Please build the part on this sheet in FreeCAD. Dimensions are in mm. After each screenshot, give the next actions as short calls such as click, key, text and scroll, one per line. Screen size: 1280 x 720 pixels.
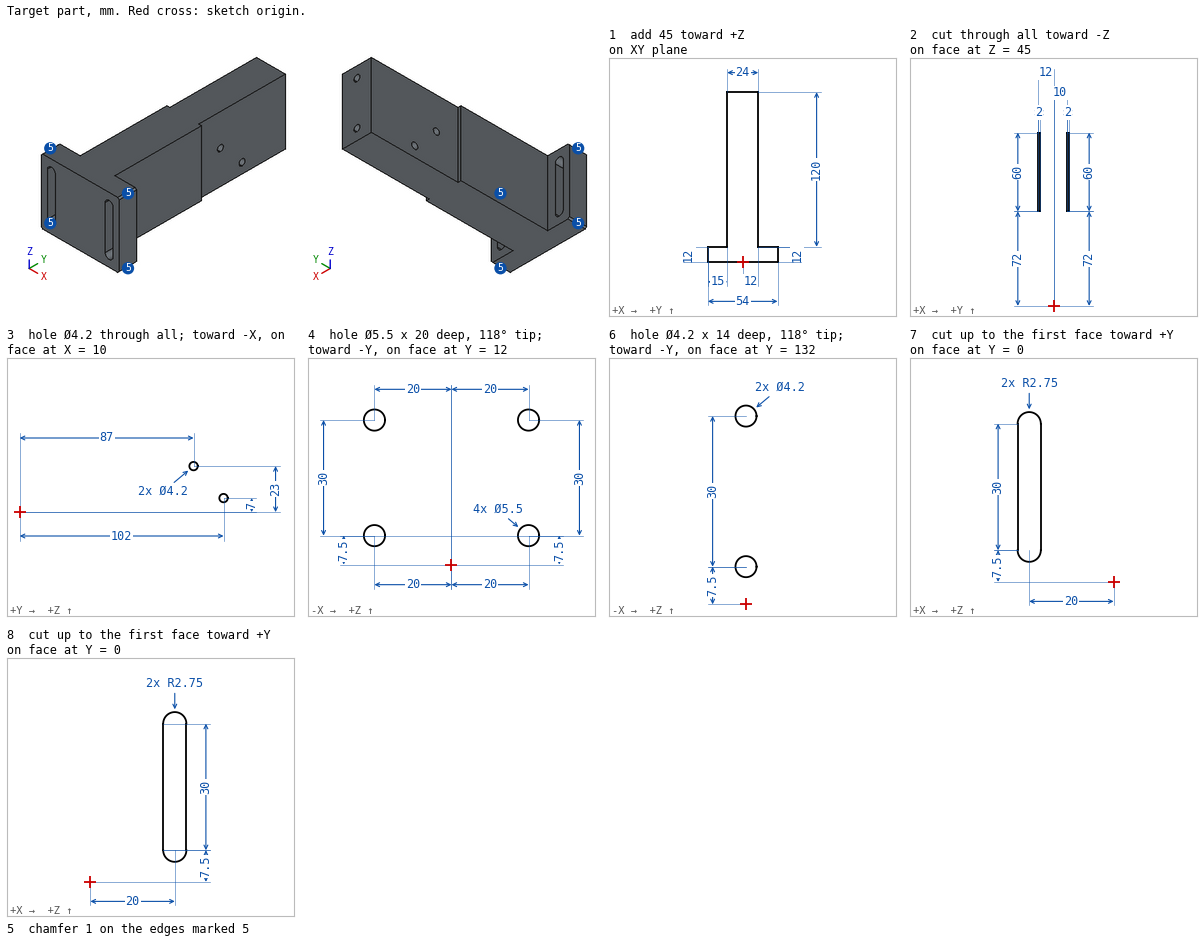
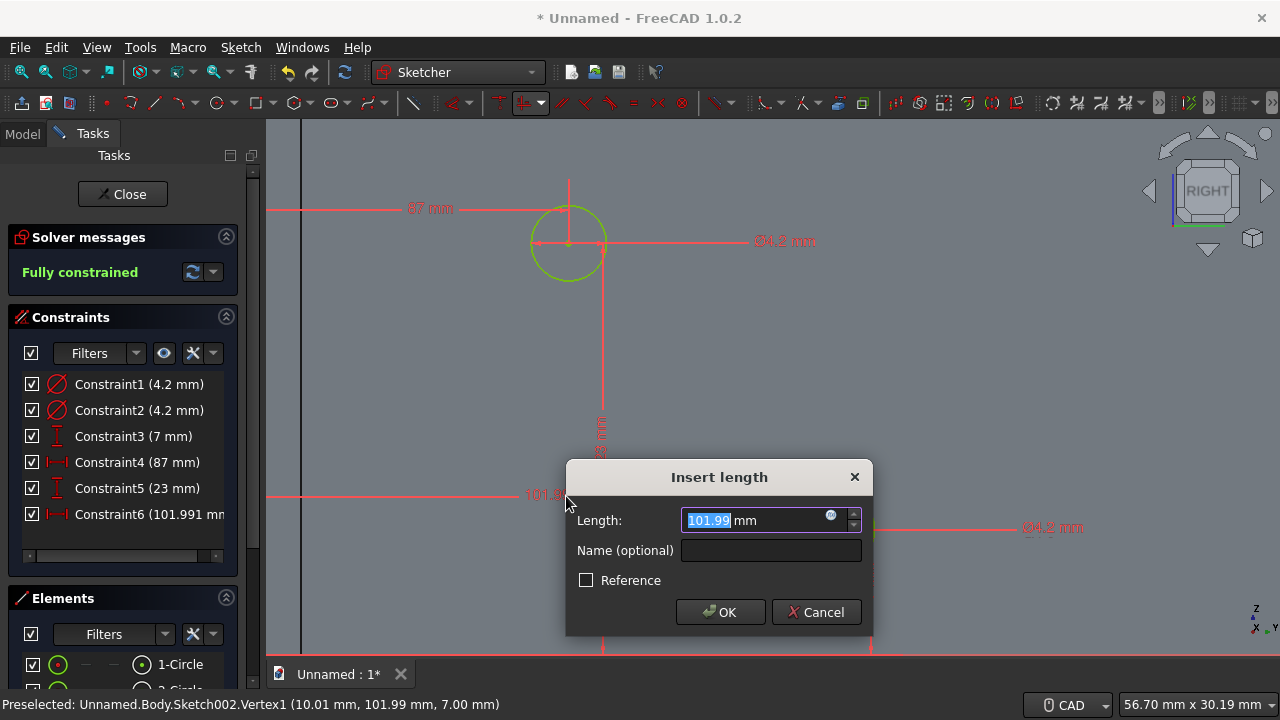
text(102)
key(Return)
key(Escape)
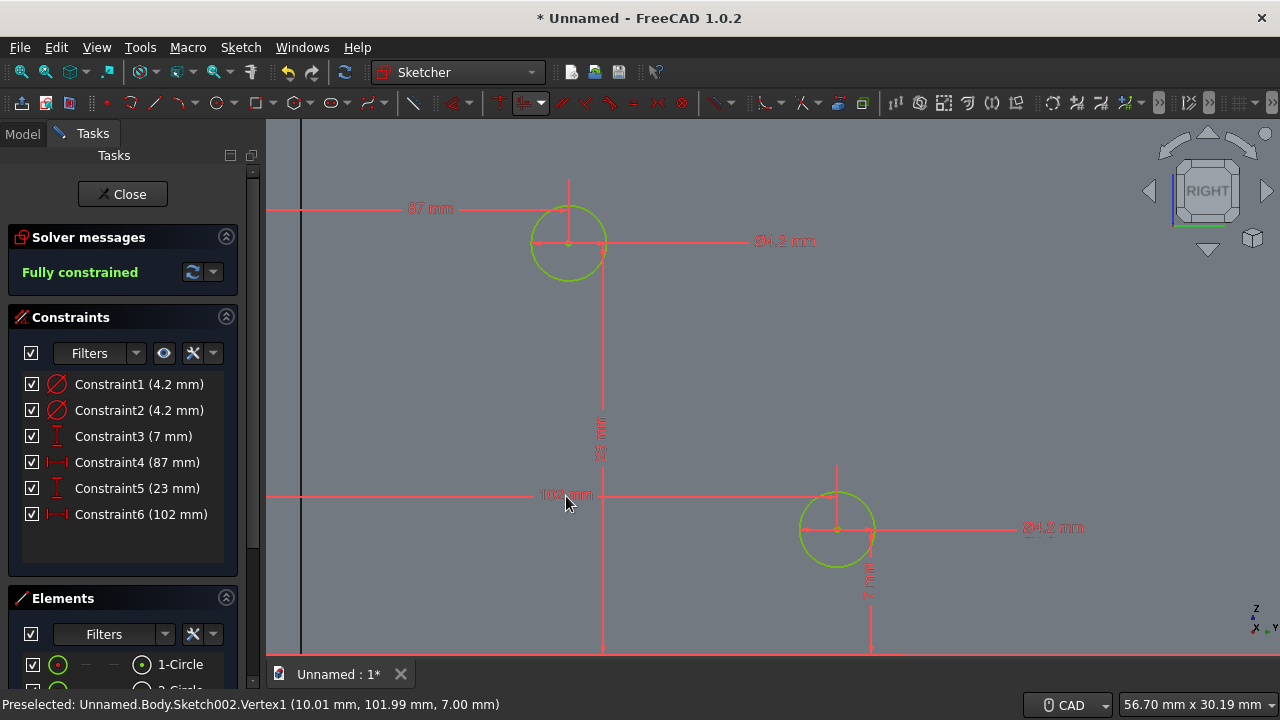
click(123, 194)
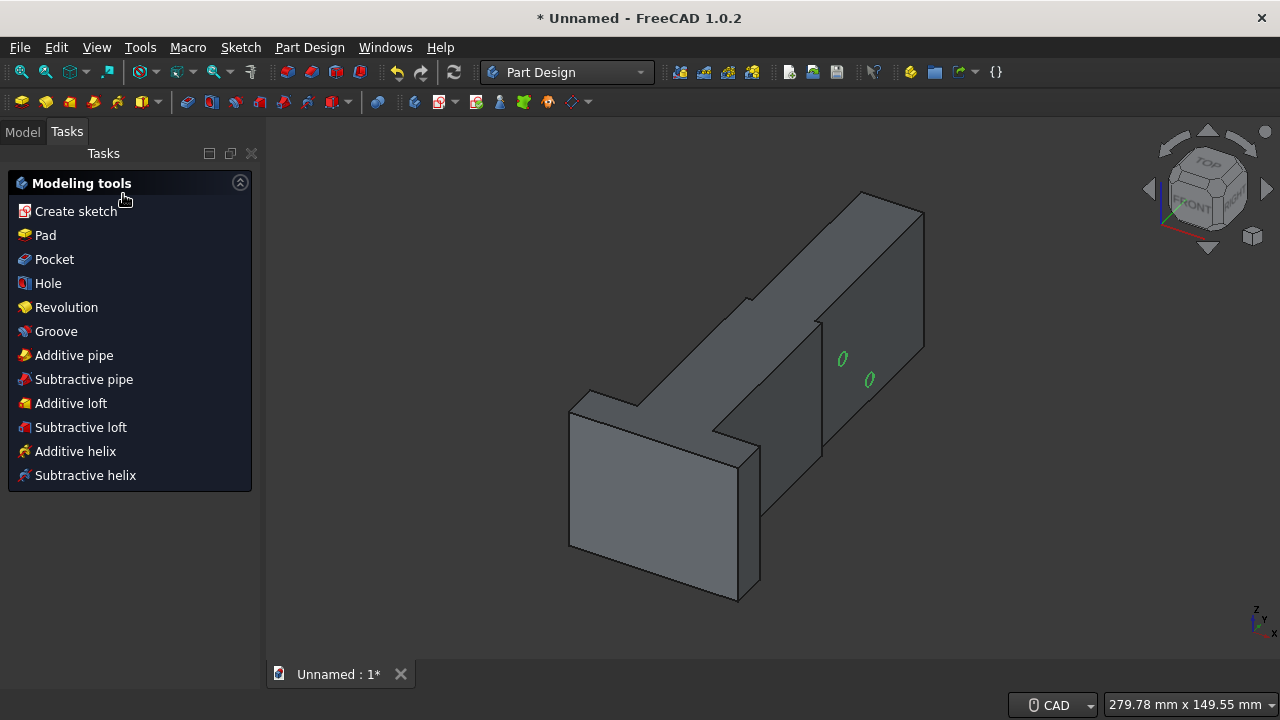
click(212, 102)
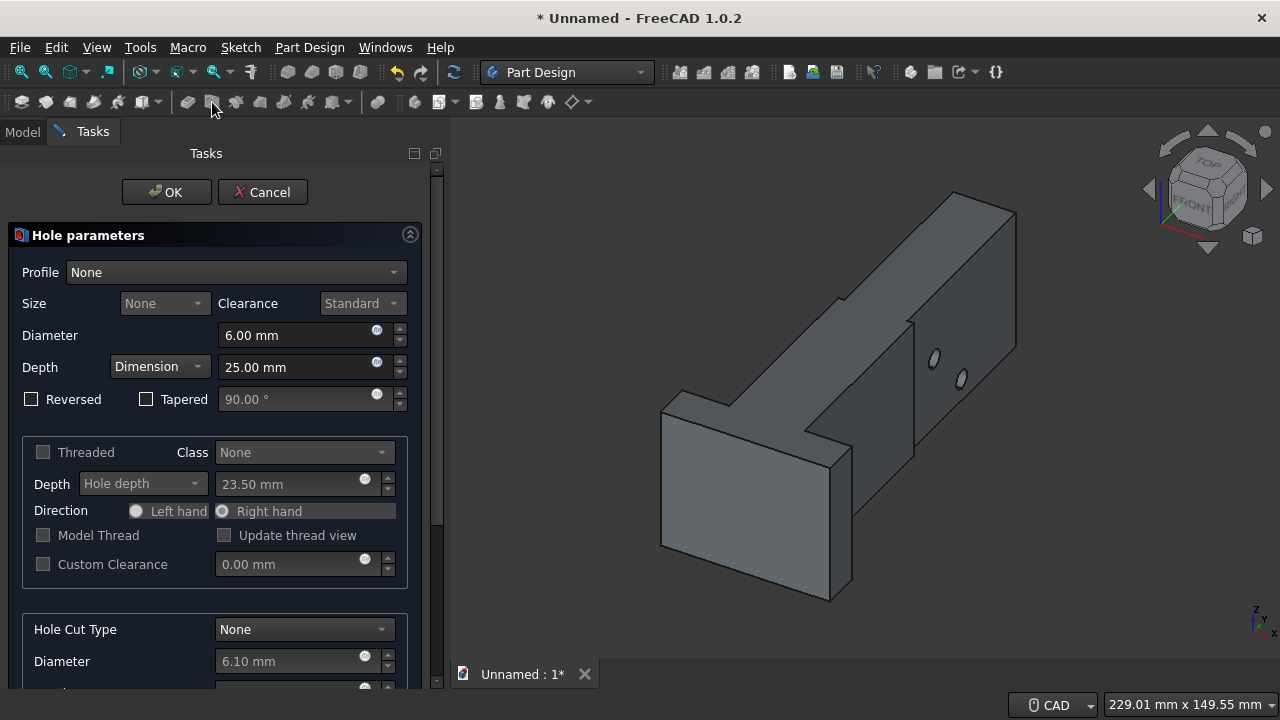
triple_click(305, 335)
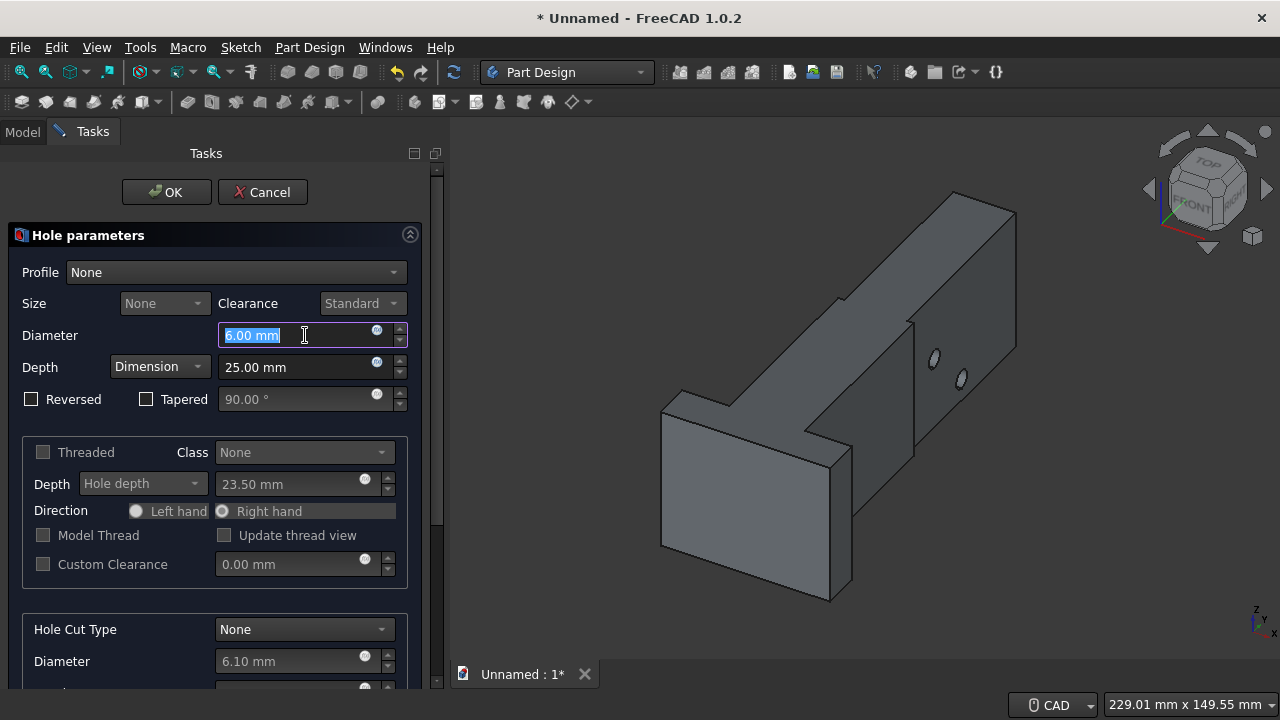
text(4.2)
key(Tab)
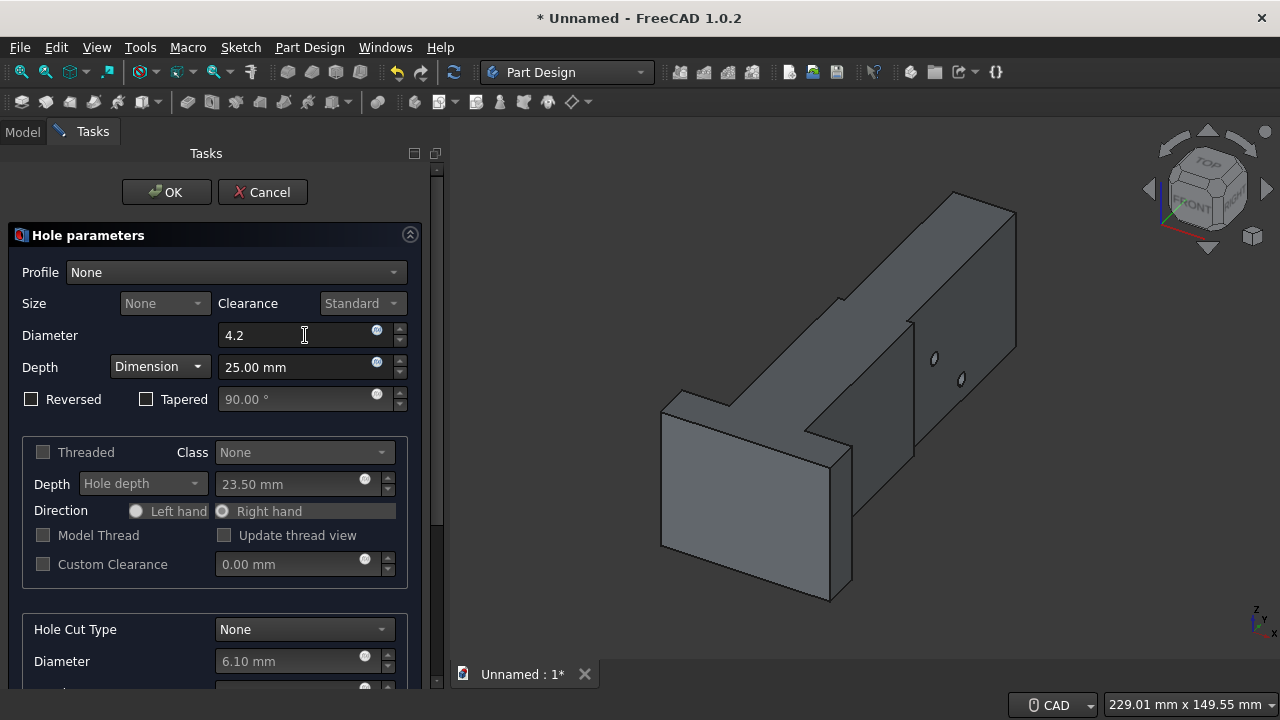
click(161, 366)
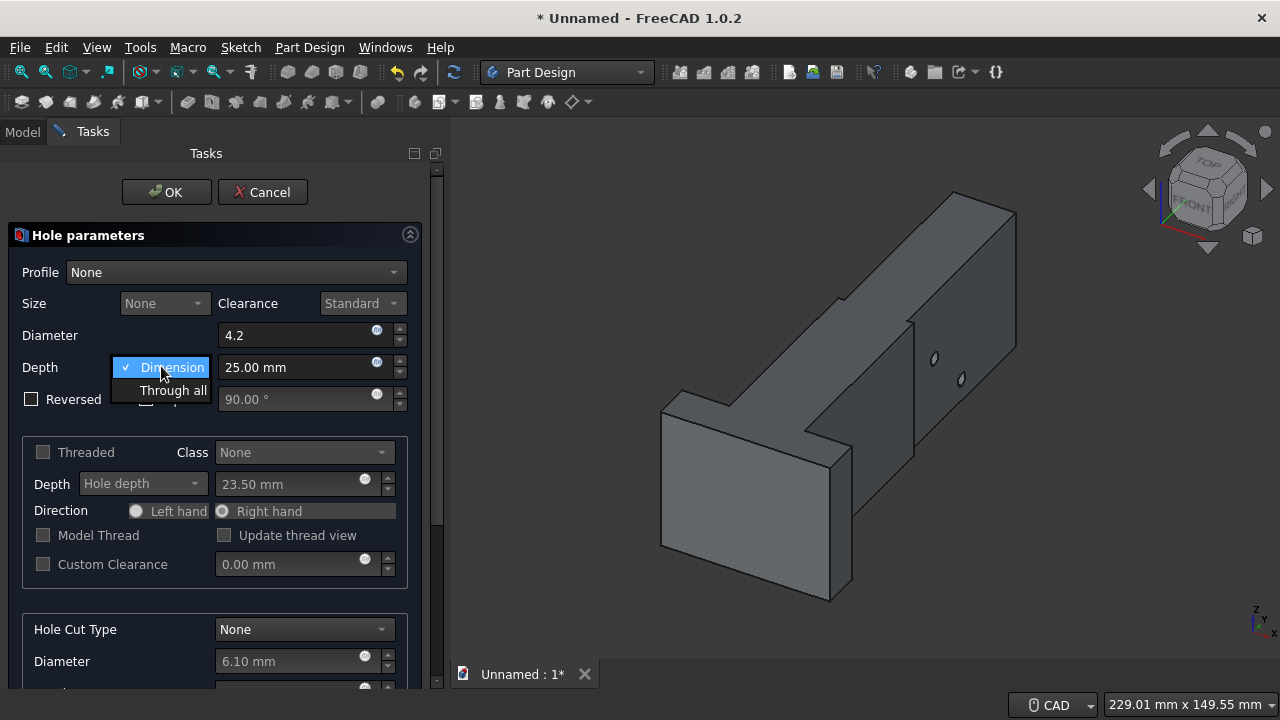
click(160, 390)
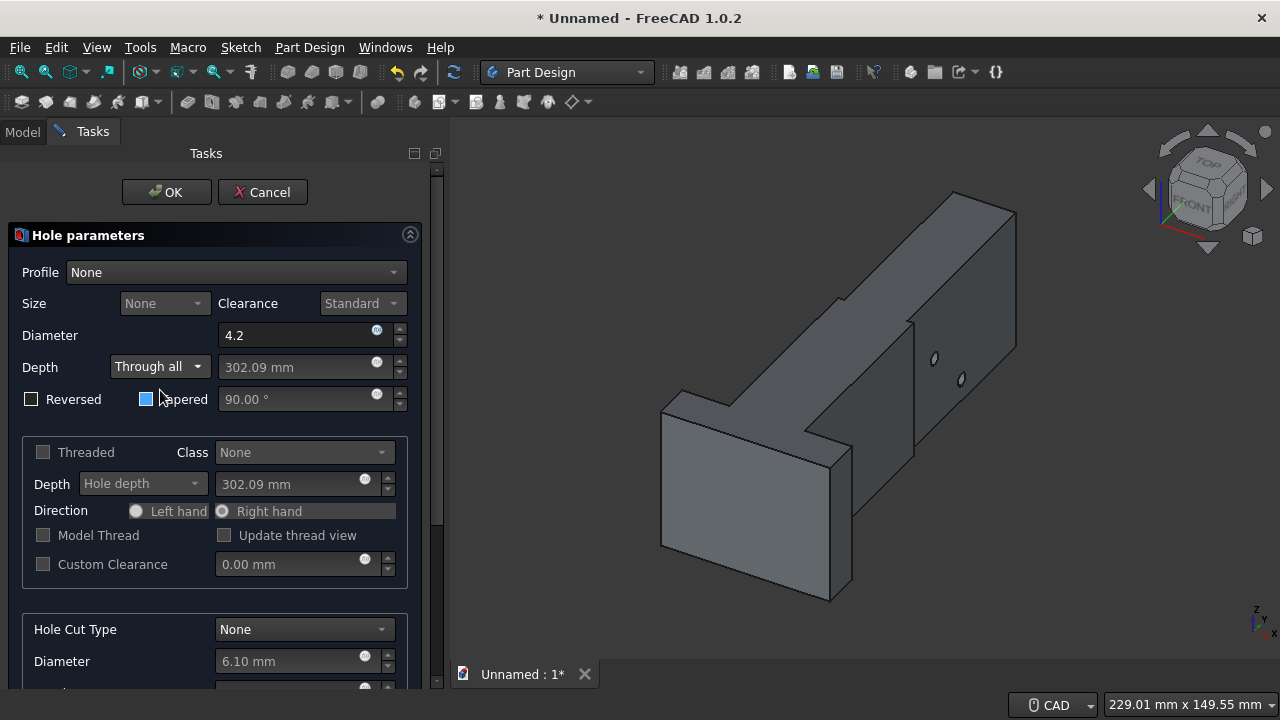
click(167, 192)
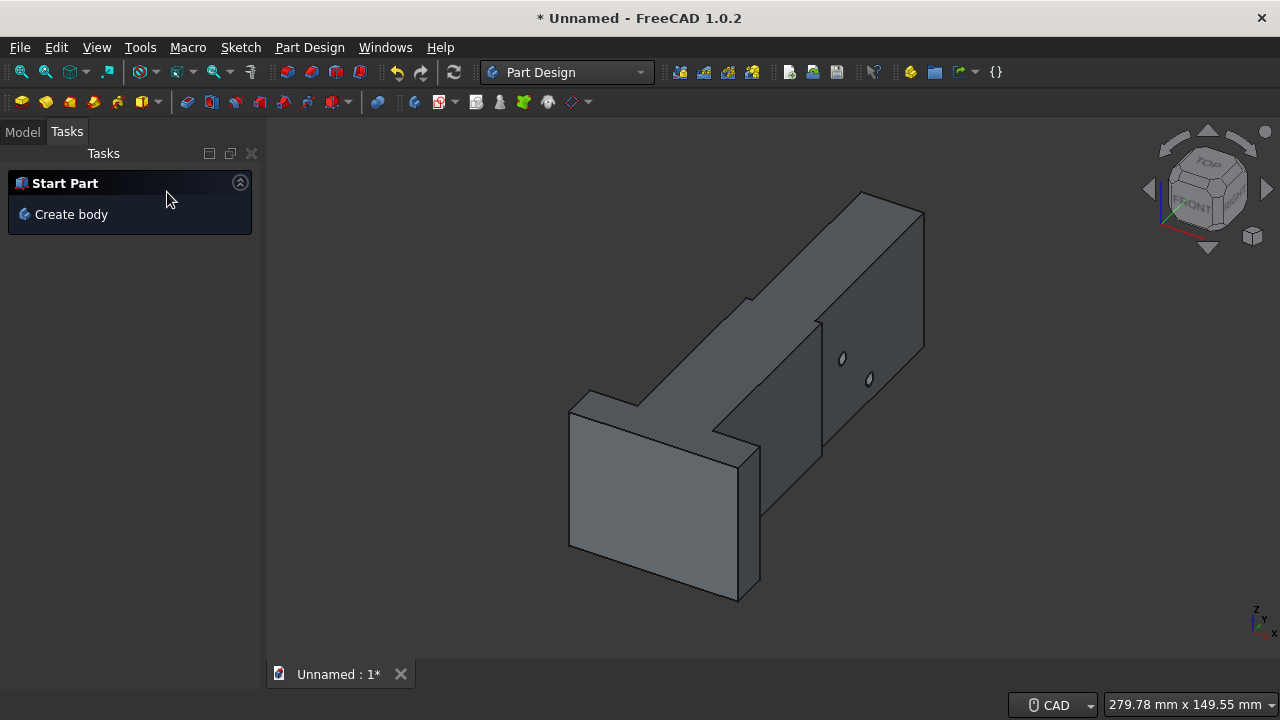
key(4)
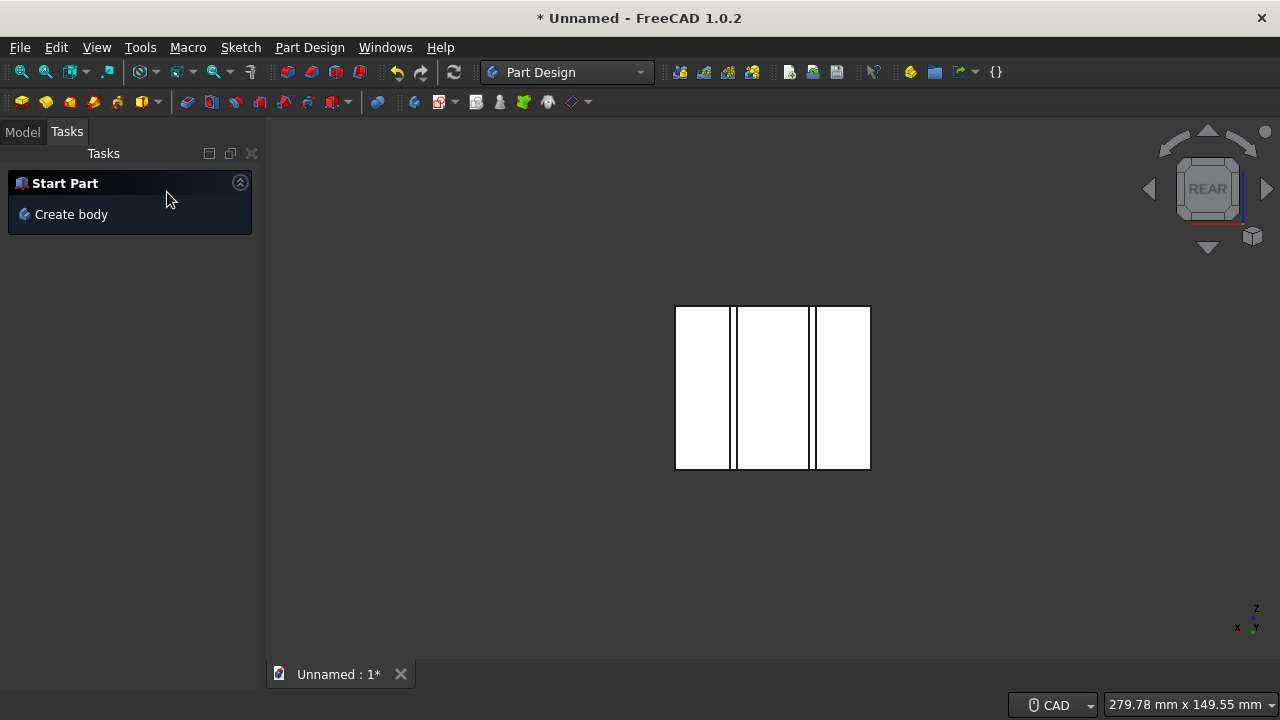
click(22, 72)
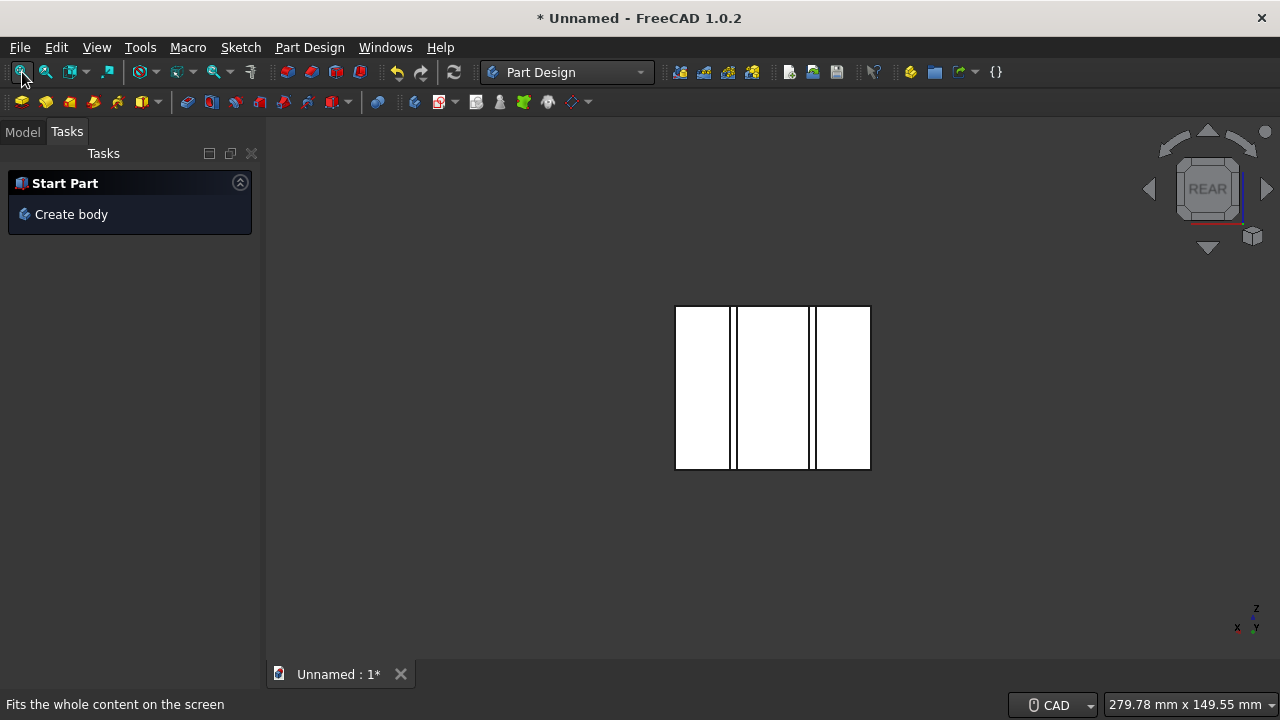
click(844, 340)